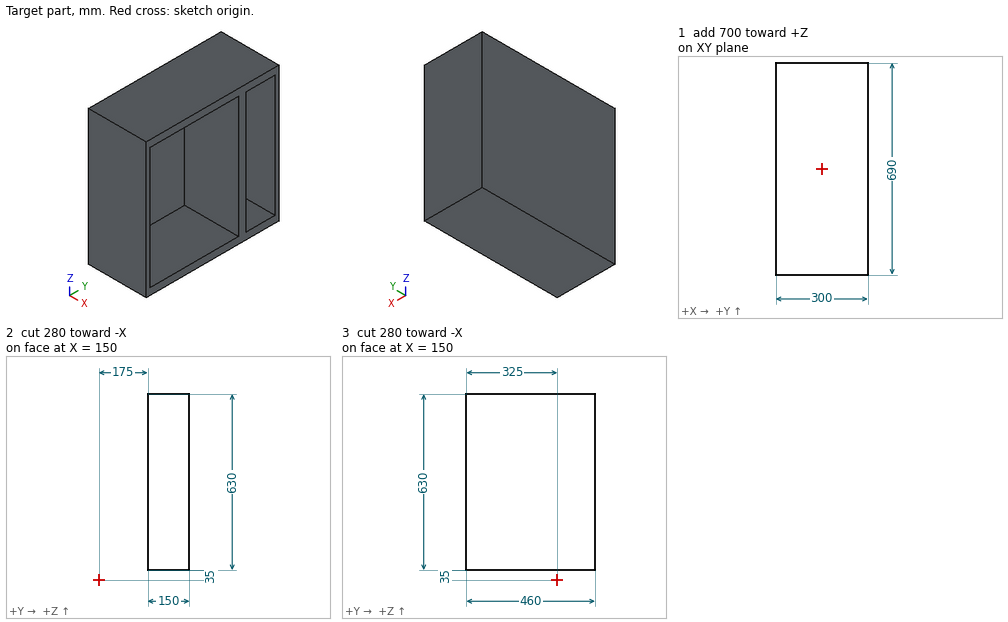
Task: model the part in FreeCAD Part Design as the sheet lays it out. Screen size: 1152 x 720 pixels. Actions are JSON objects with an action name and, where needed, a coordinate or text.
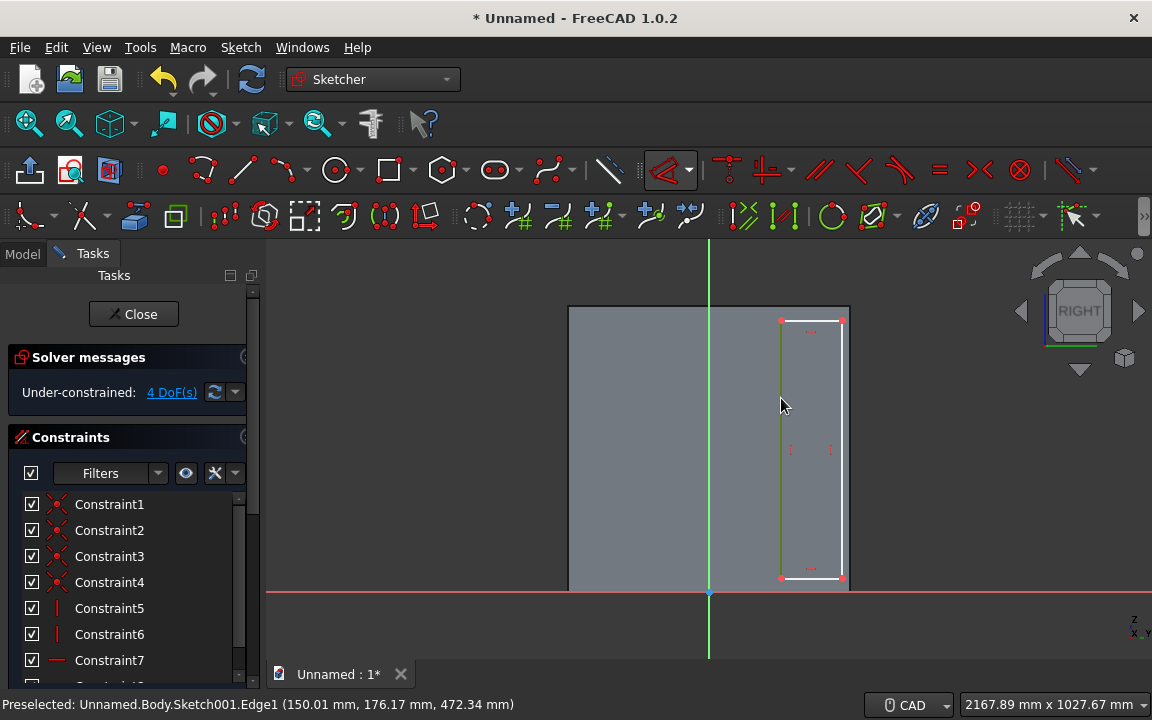
{"action": "key", "text": "i"}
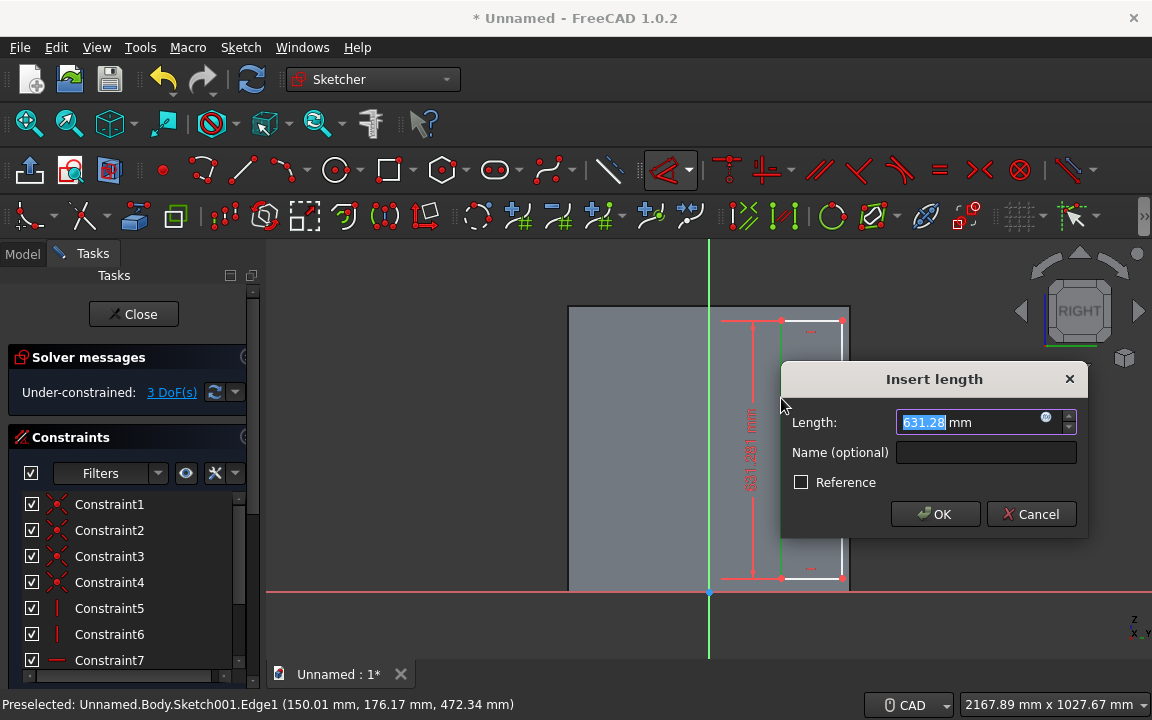
{"action": "type", "text": "630"}
{"action": "key", "text": "Return"}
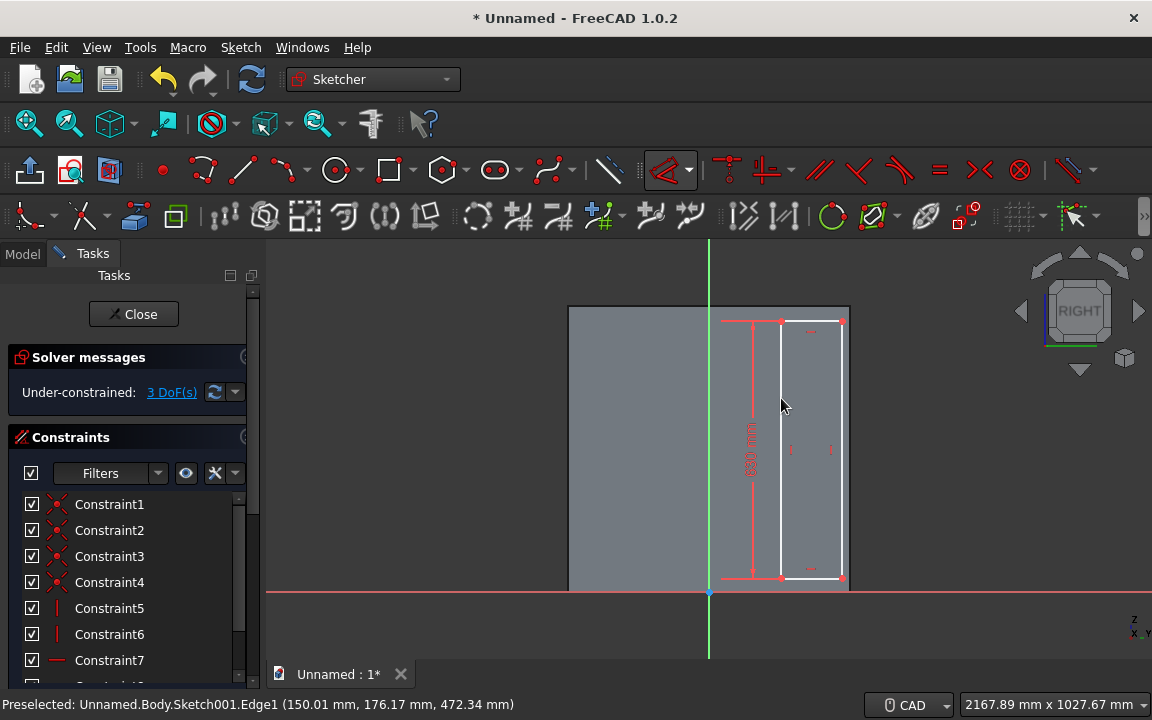
{"action": "left_click", "coordinate": [799, 579]}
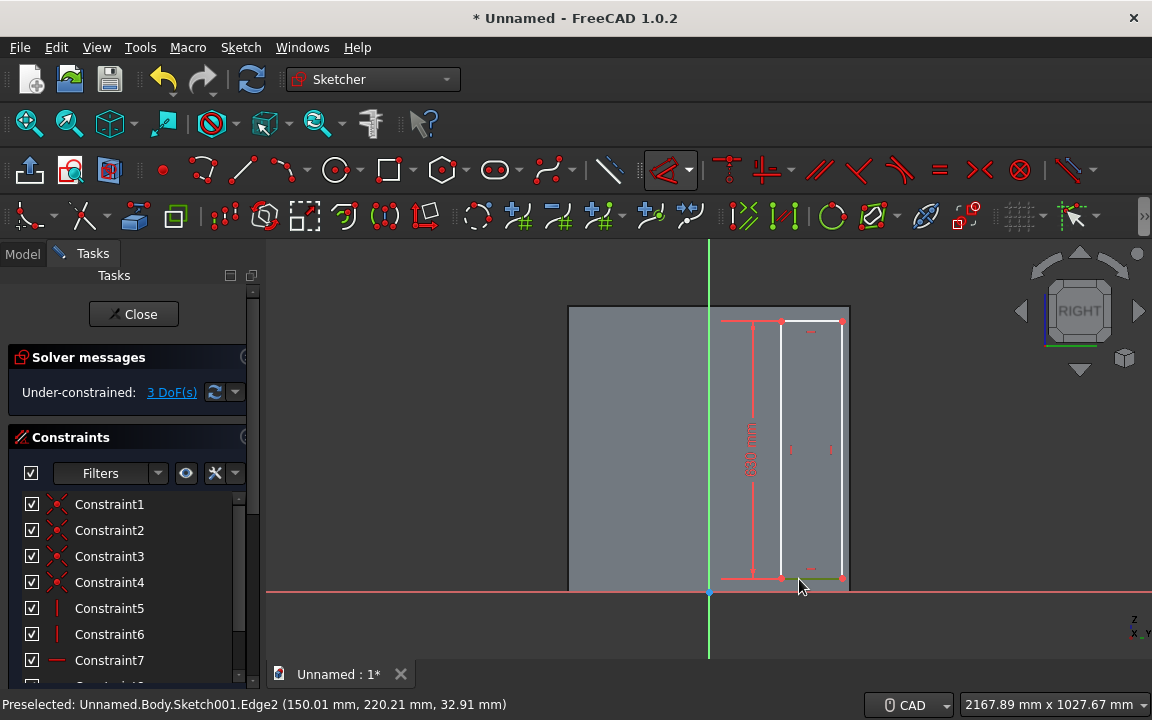
{"action": "key", "text": "l"}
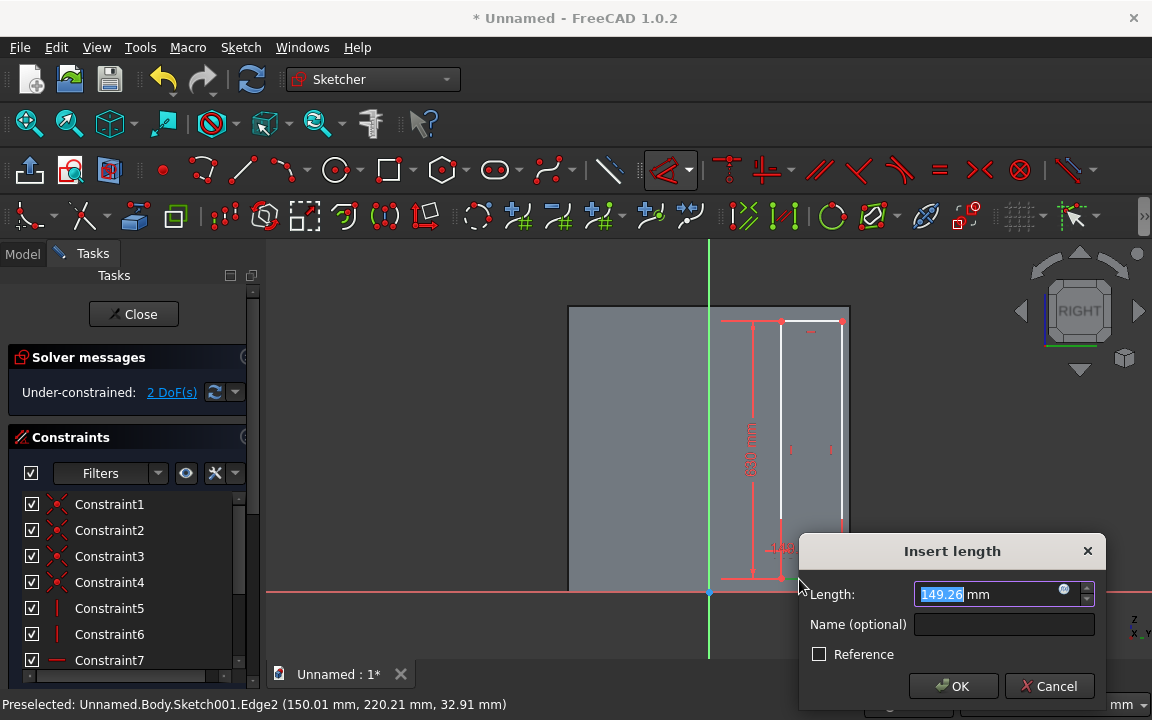
{"action": "type", "text": "150"}
{"action": "key", "text": "Return"}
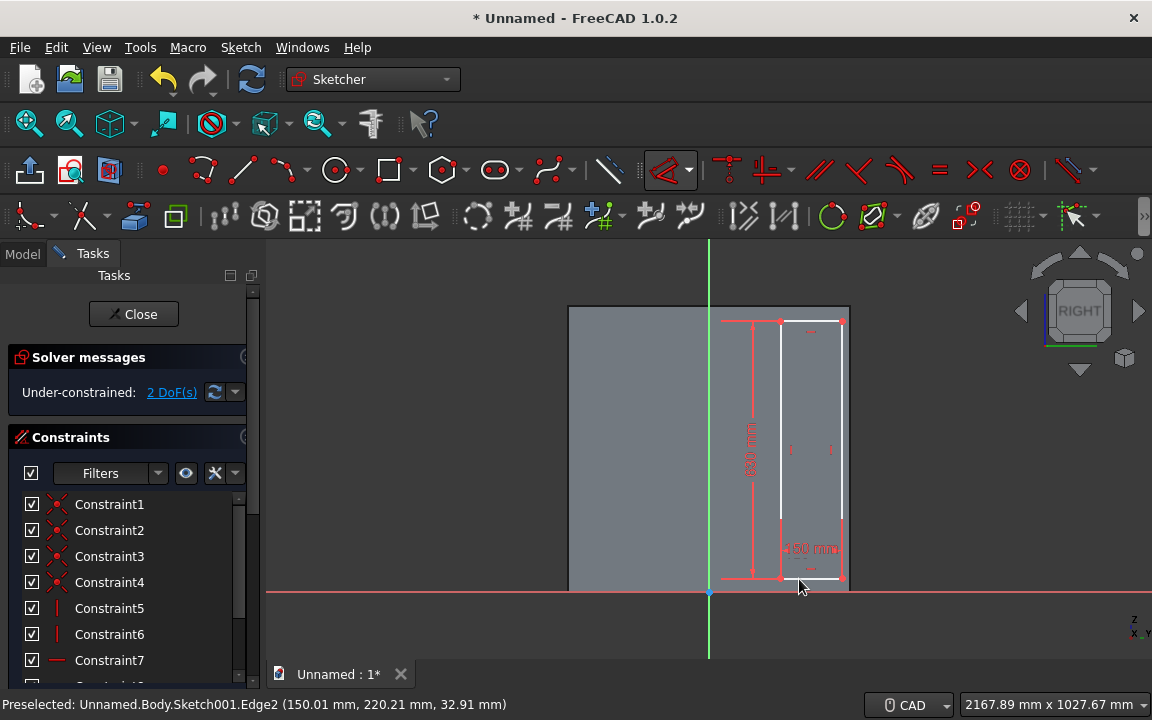
{"action": "scroll", "coordinate": [781, 579], "scroll_direction": "up", "scroll_amount": 6}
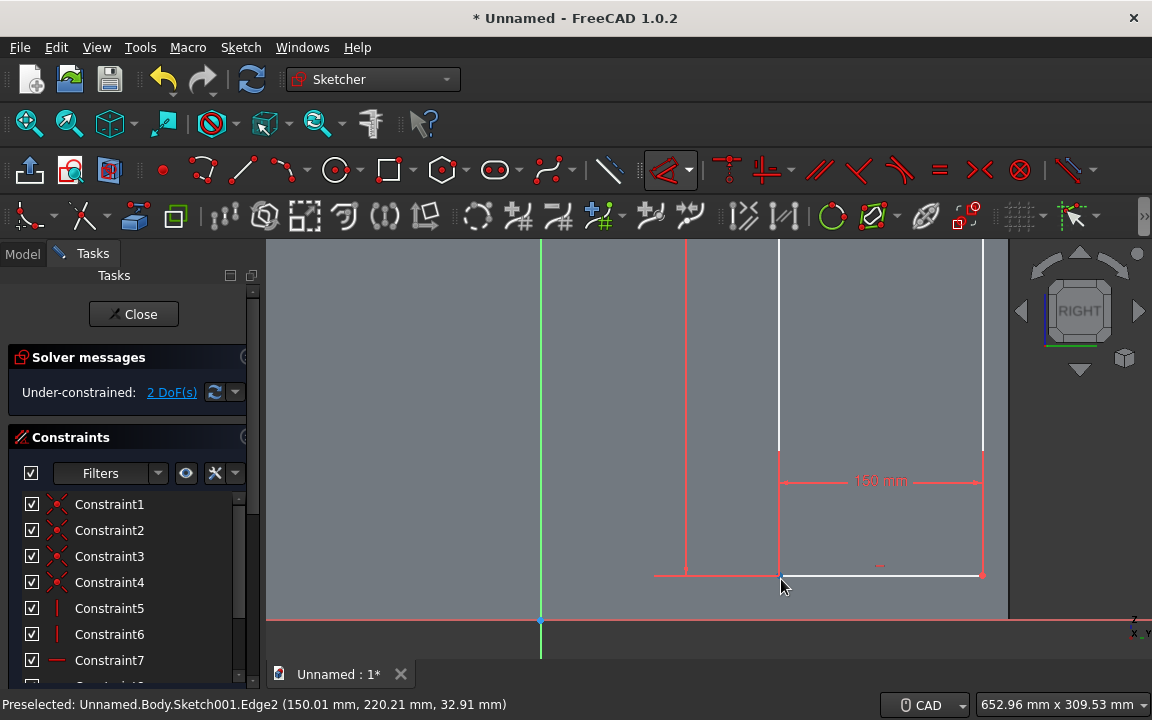
{"action": "left_click", "coordinate": [779, 576]}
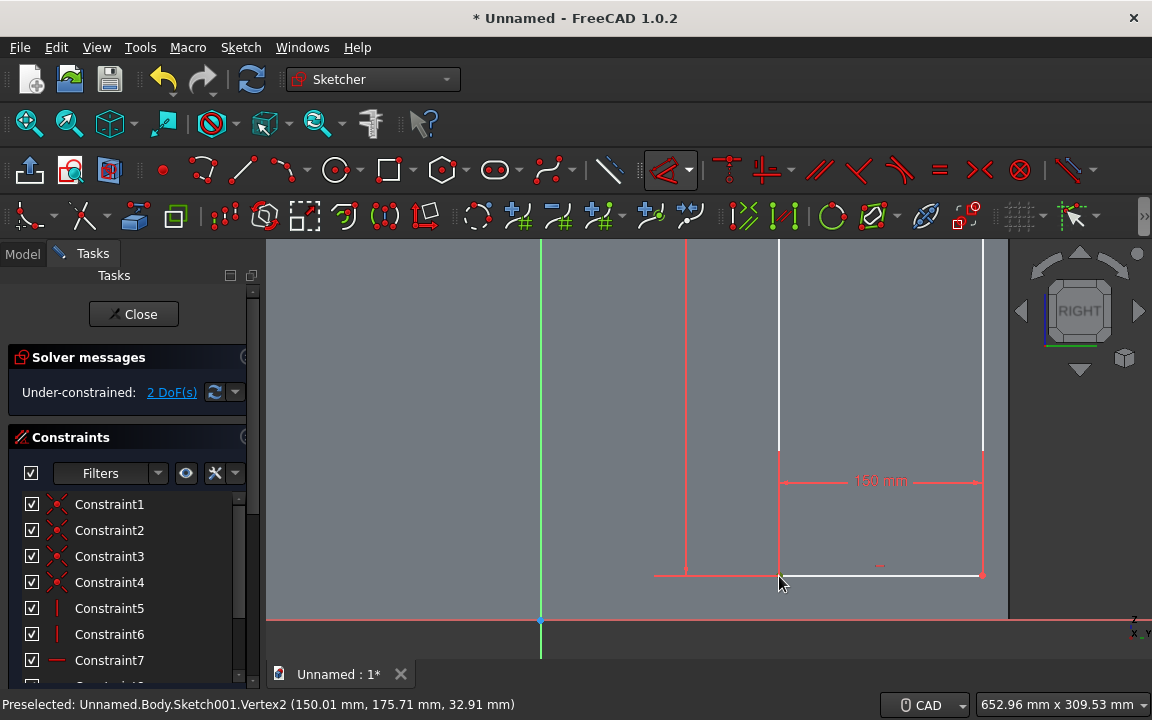
{"action": "key", "text": "i"}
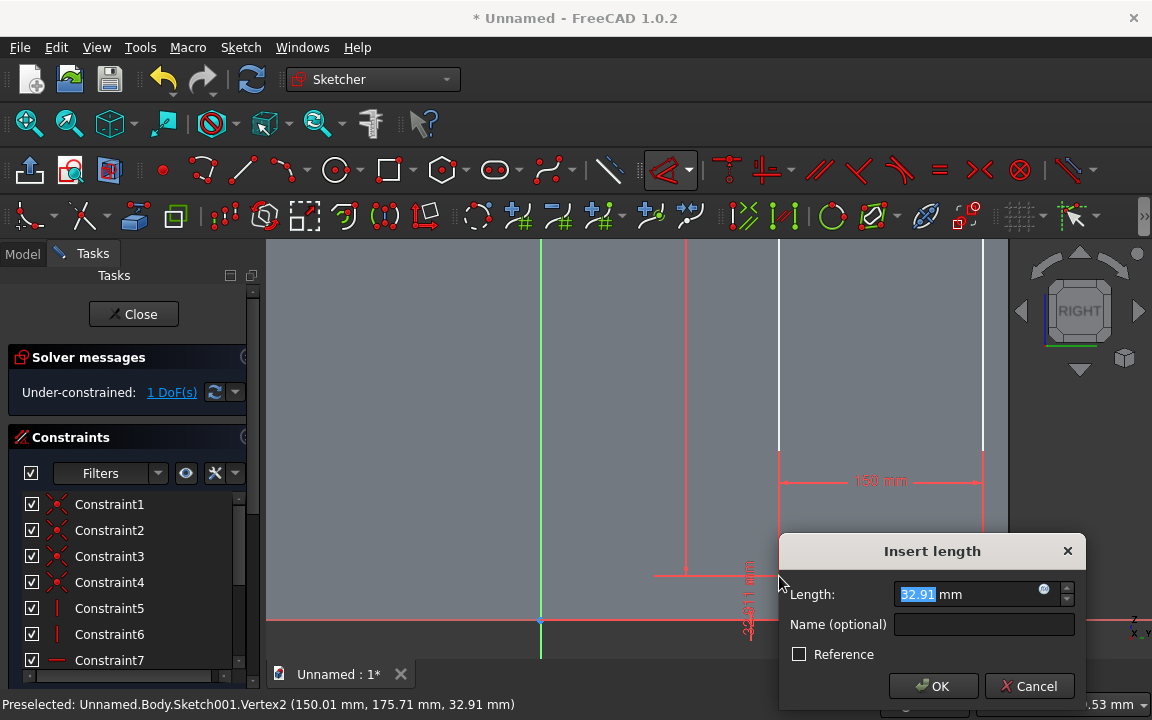
{"action": "type", "text": "35"}
{"action": "key", "text": "Return"}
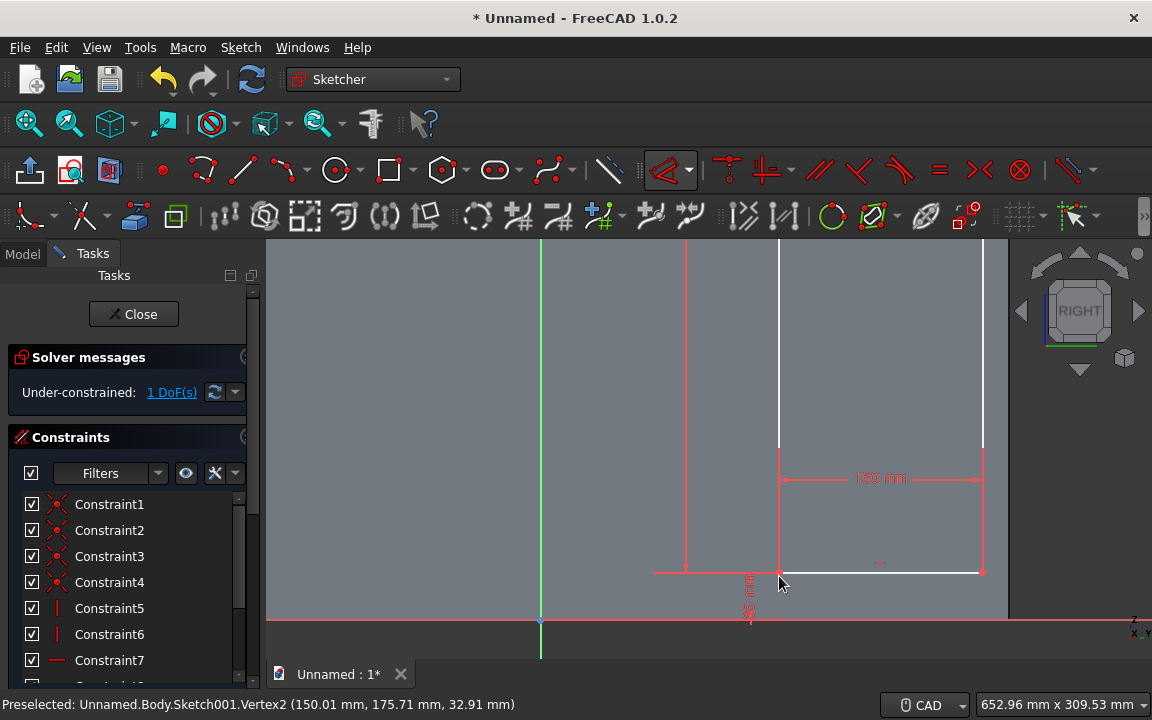
{"action": "scroll", "coordinate": [589, 570], "scroll_direction": "down", "scroll_amount": 6}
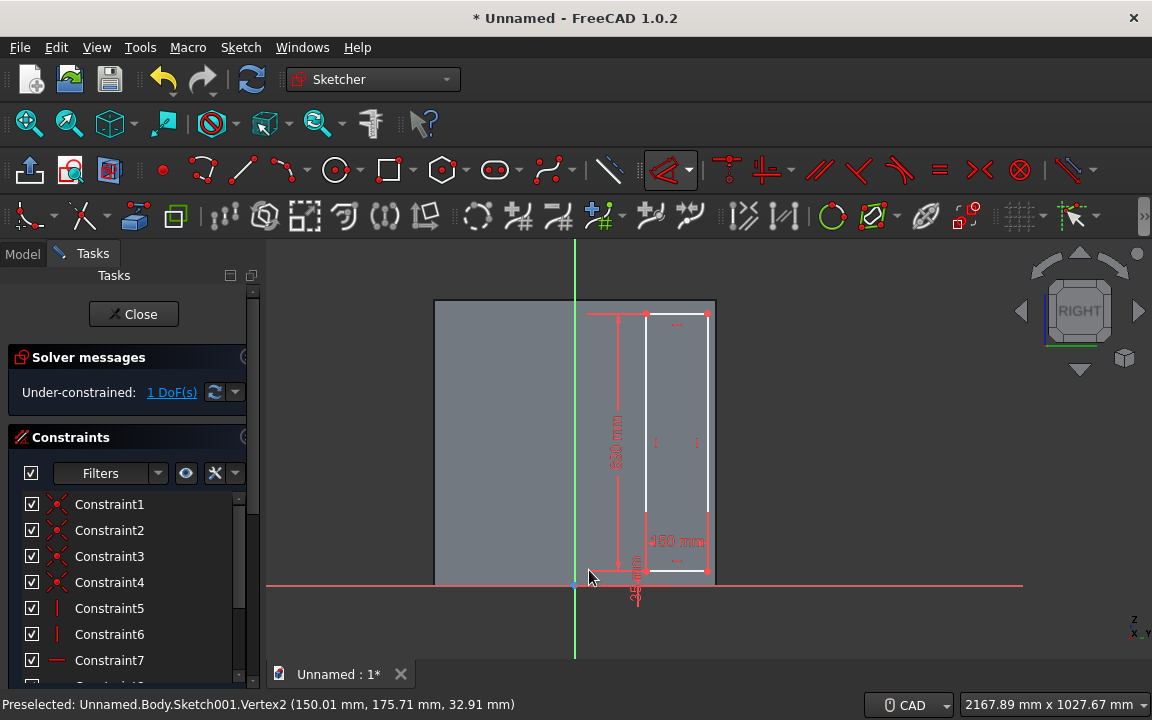
{"action": "left_click", "coordinate": [646, 314]}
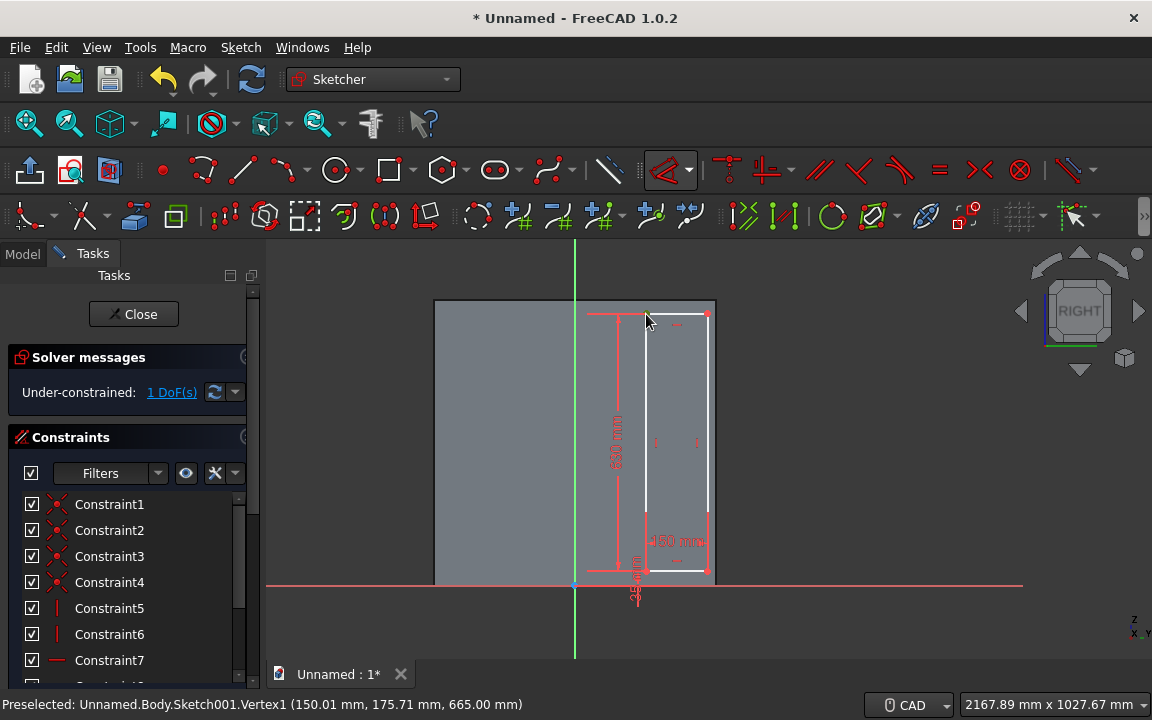
{"action": "key", "text": "l"}